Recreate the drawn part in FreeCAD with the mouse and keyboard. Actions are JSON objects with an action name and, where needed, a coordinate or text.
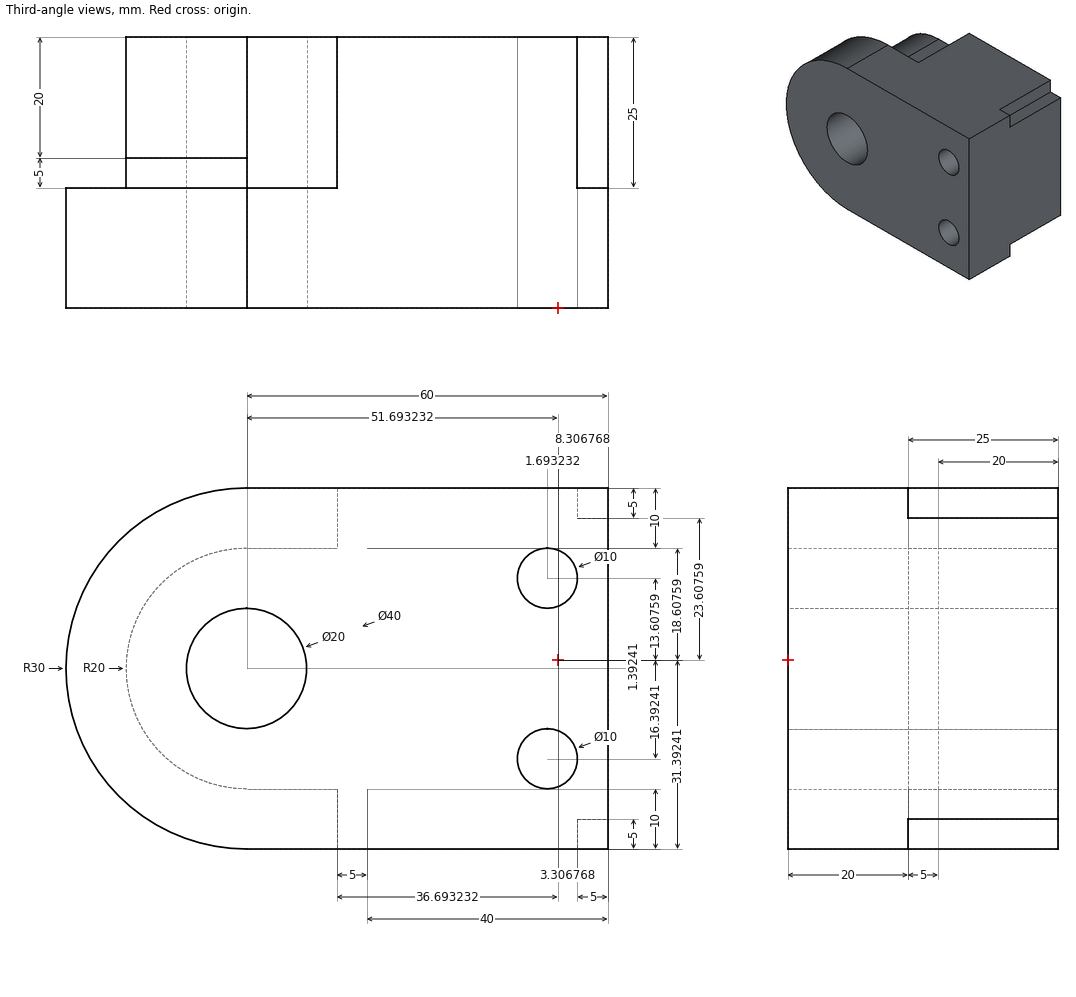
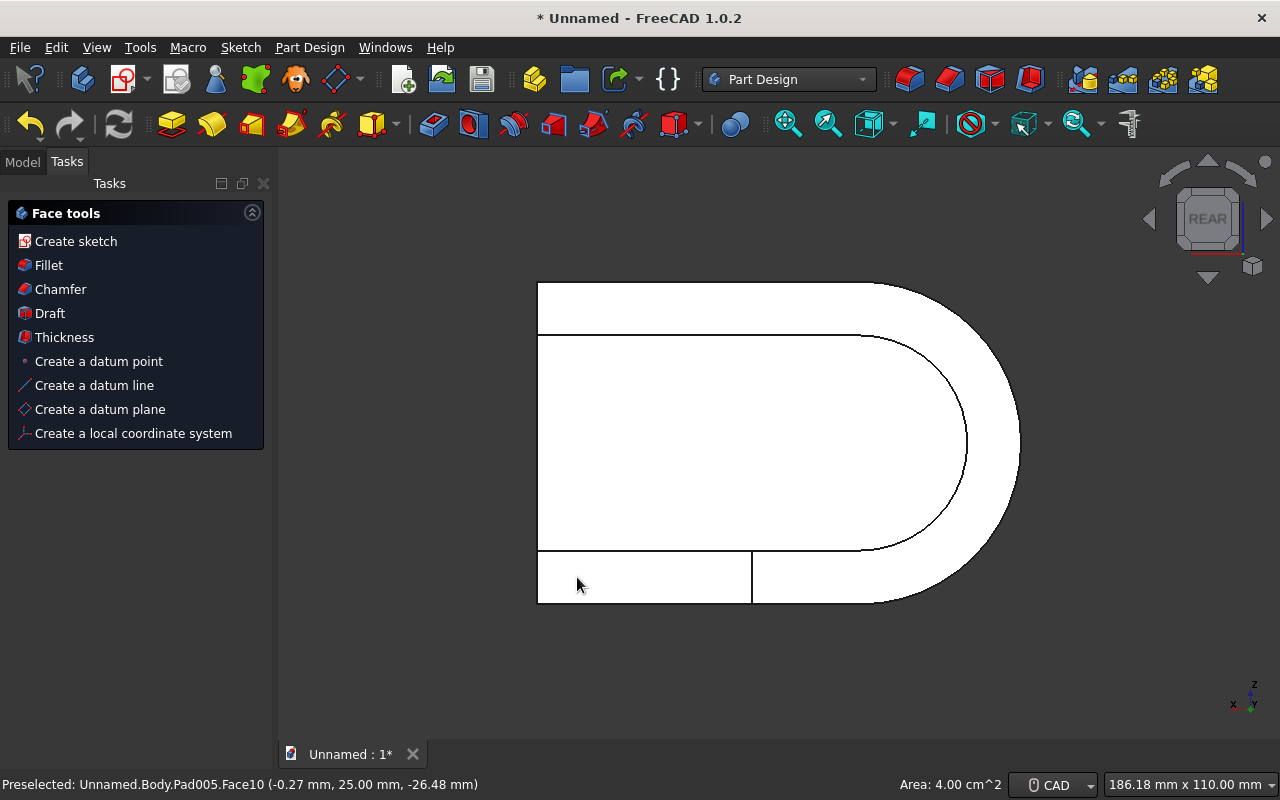
{"action": "left_click", "coordinate": [124, 80]}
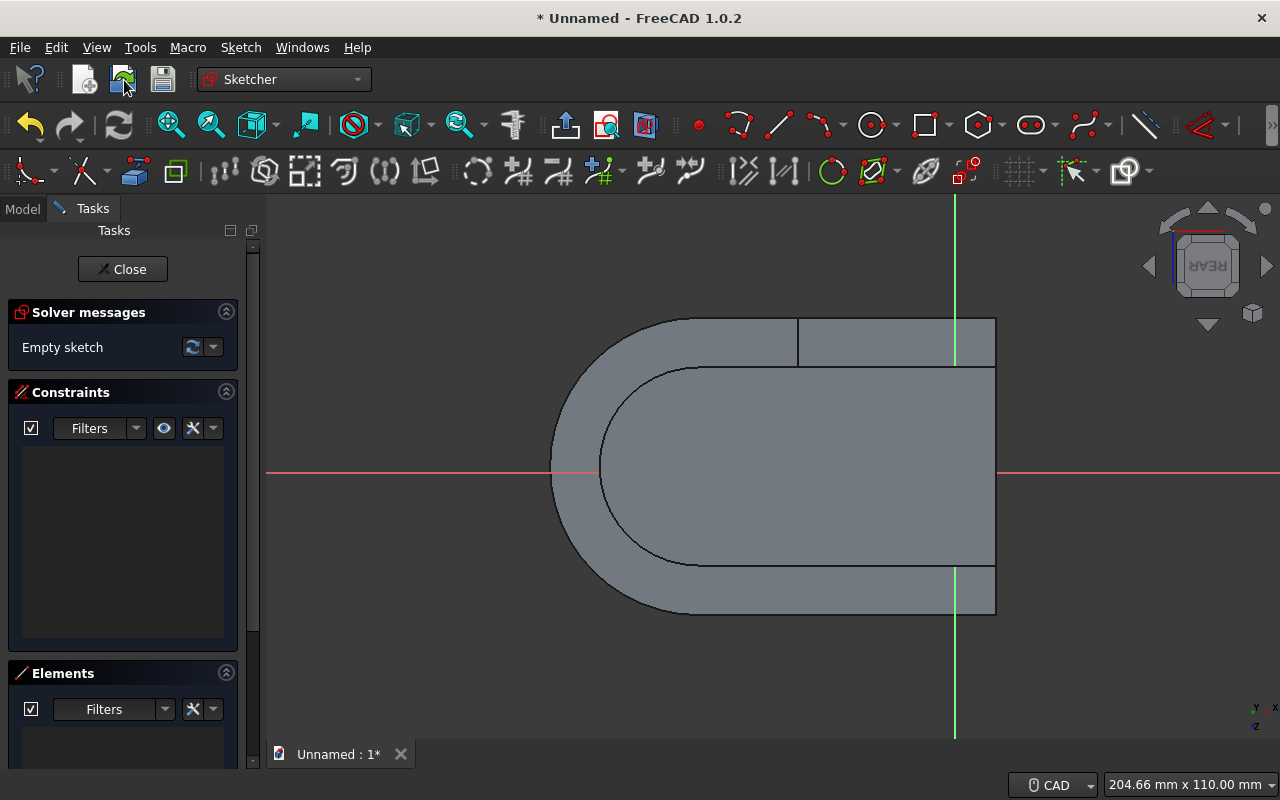
{"action": "left_click", "coordinate": [646, 126]}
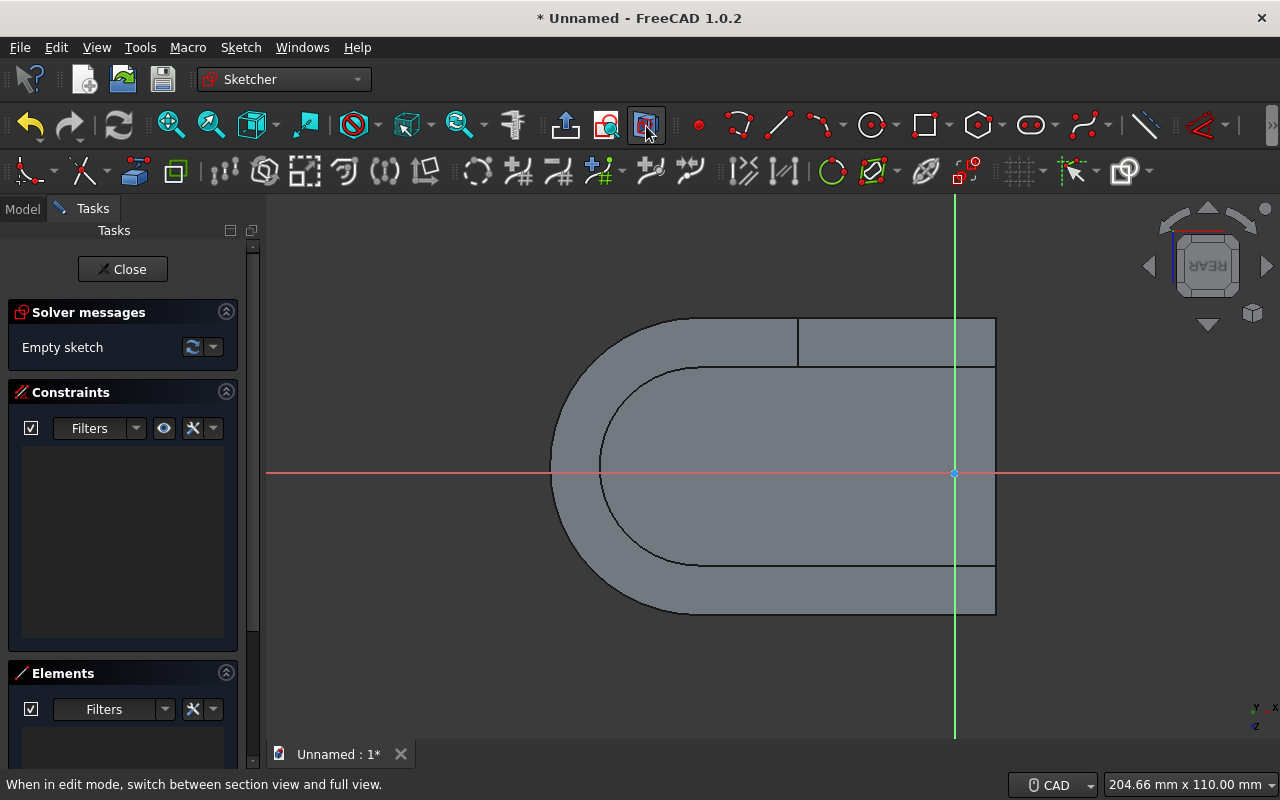
{"action": "scroll", "coordinate": [1054, 338], "scroll_direction": "up", "scroll_amount": 4}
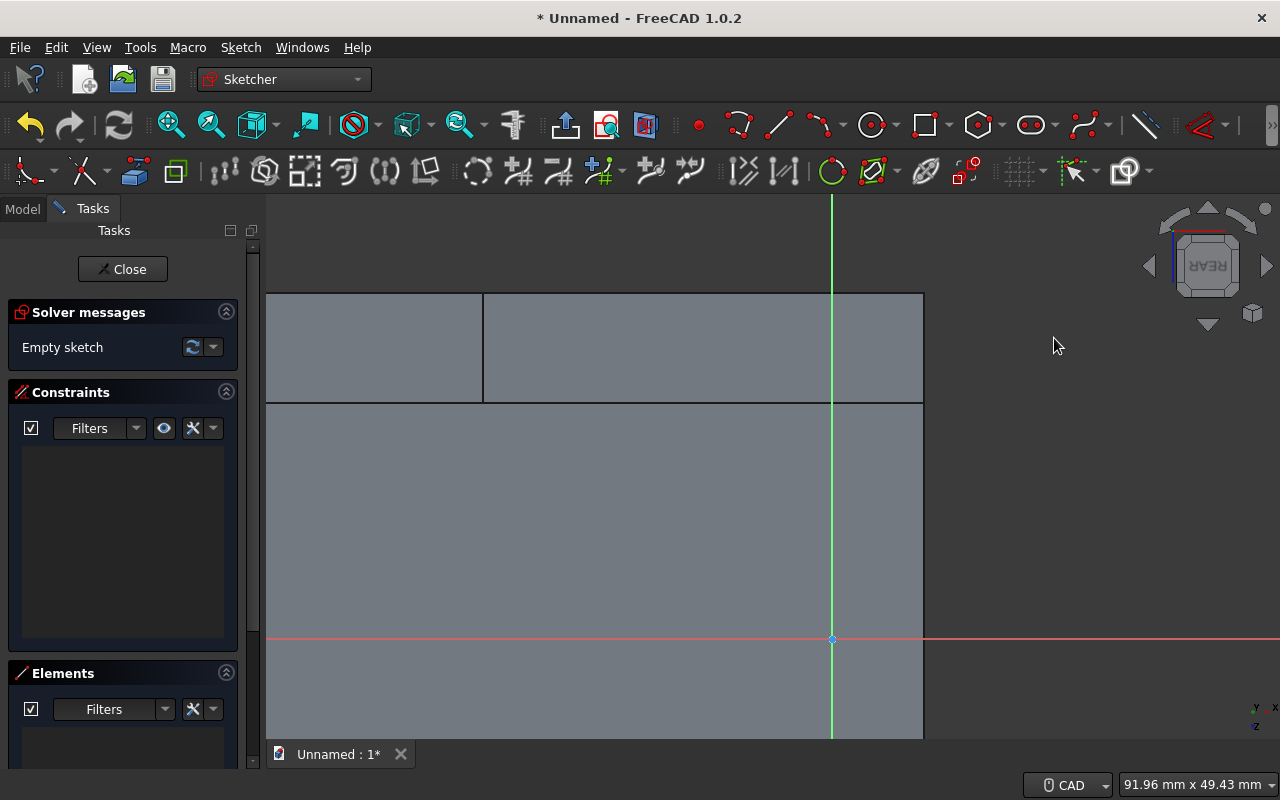
{"action": "key", "text": "g r"}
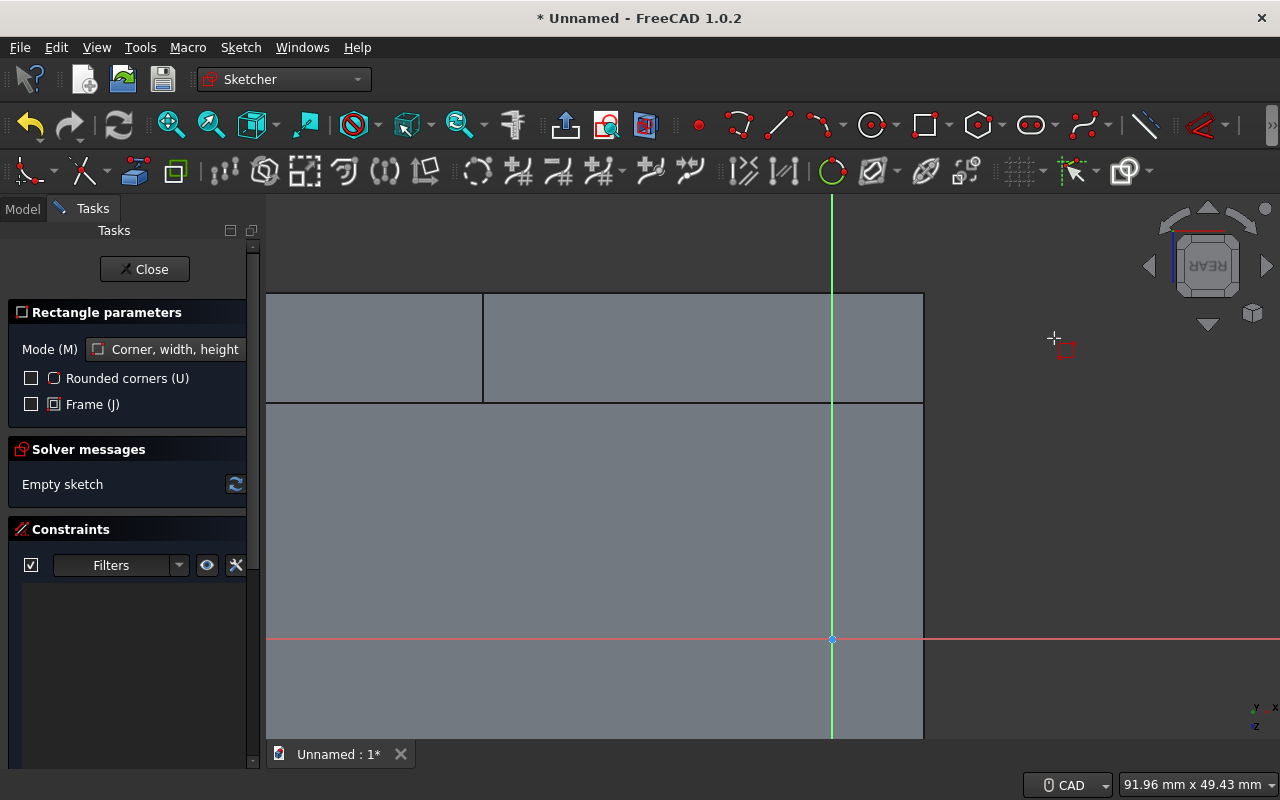
{"action": "left_click", "coordinate": [483, 293]}
{"action": "left_click", "coordinate": [924, 403]}
{"action": "key", "text": "Escape"}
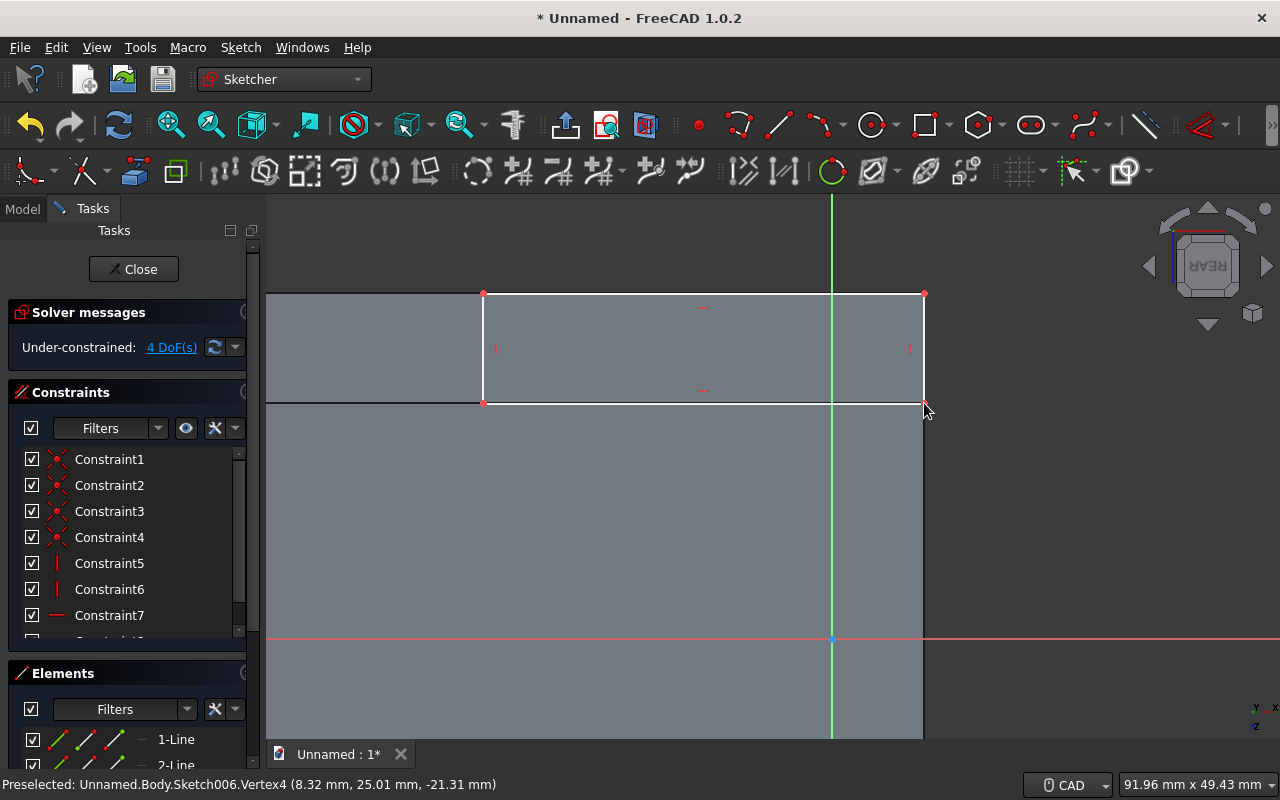
{"action": "left_click", "coordinate": [1200, 126]}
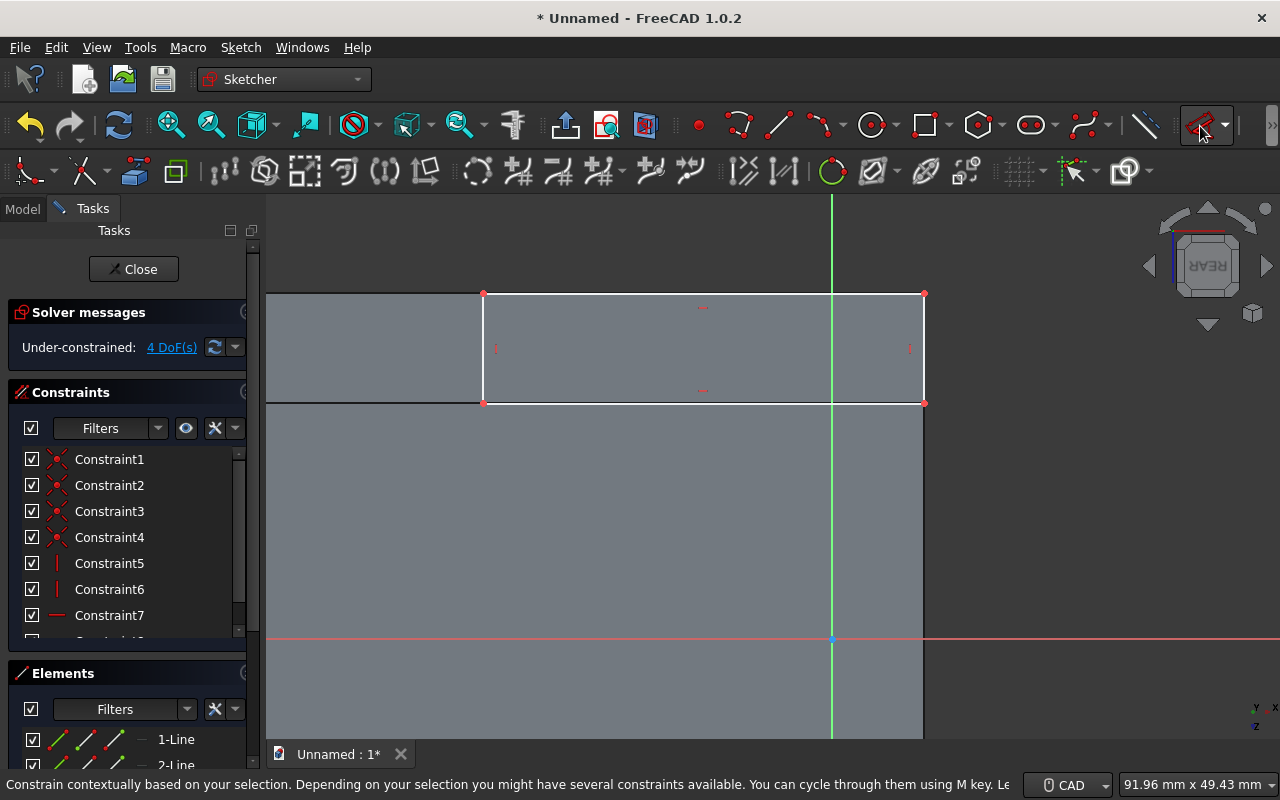
{"action": "left_click", "coordinate": [483, 327]}
{"action": "left_click", "coordinate": [449, 349]}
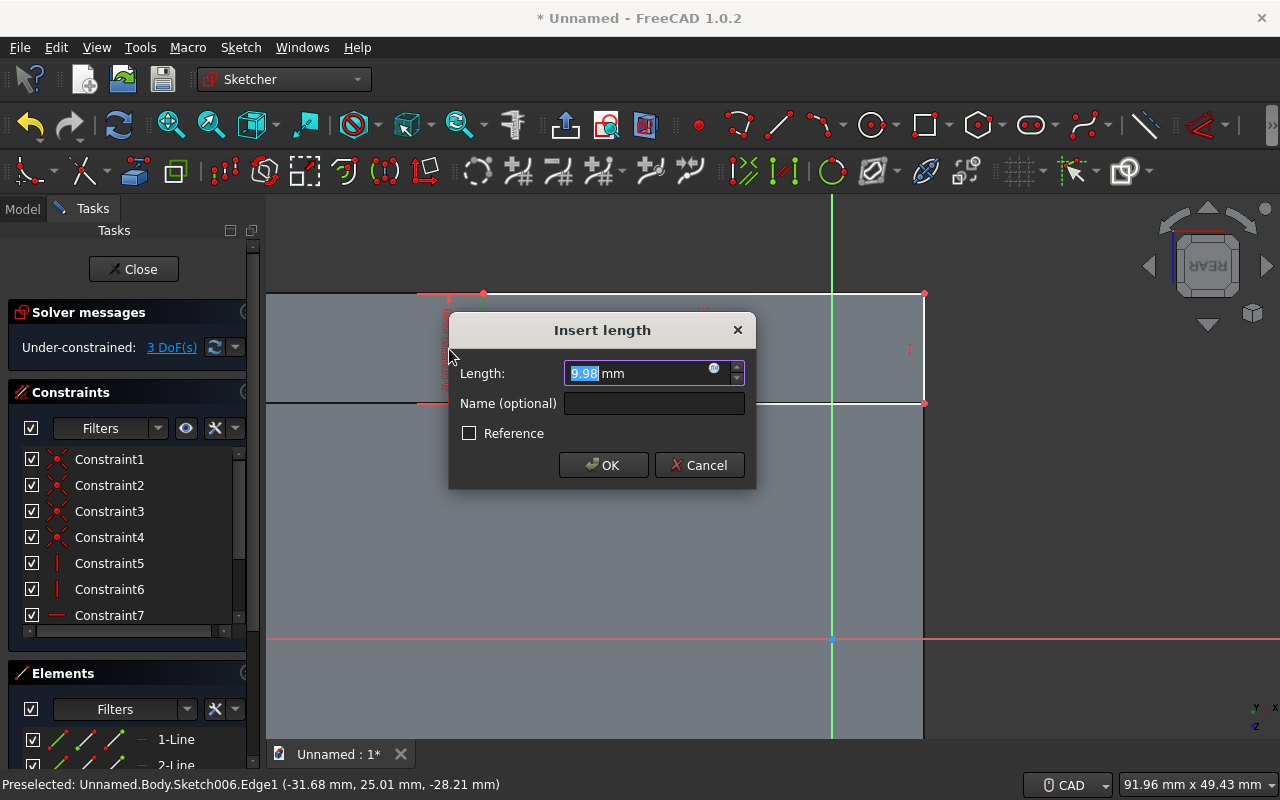
{"action": "type", "text": "10"}
{"action": "key", "text": "Return"}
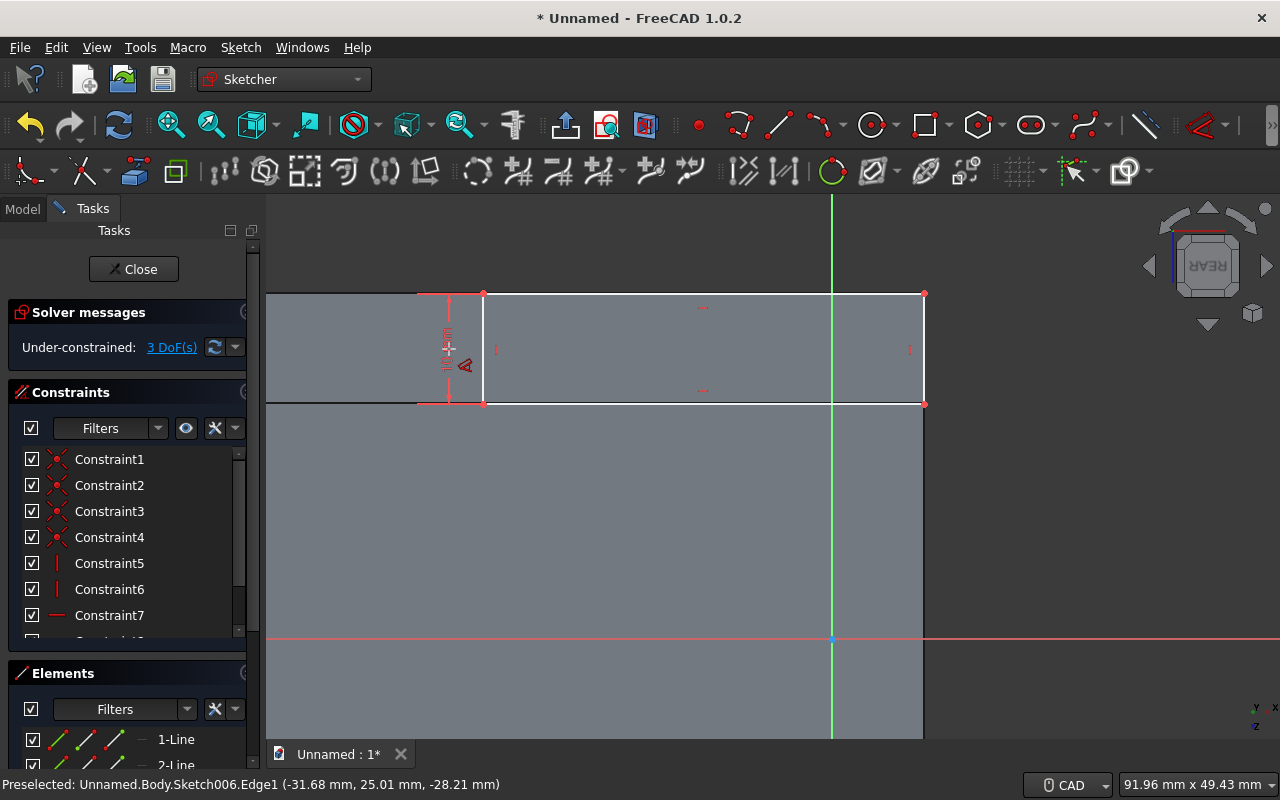
{"action": "left_click", "coordinate": [615, 404]}
{"action": "left_click", "coordinate": [703, 370]}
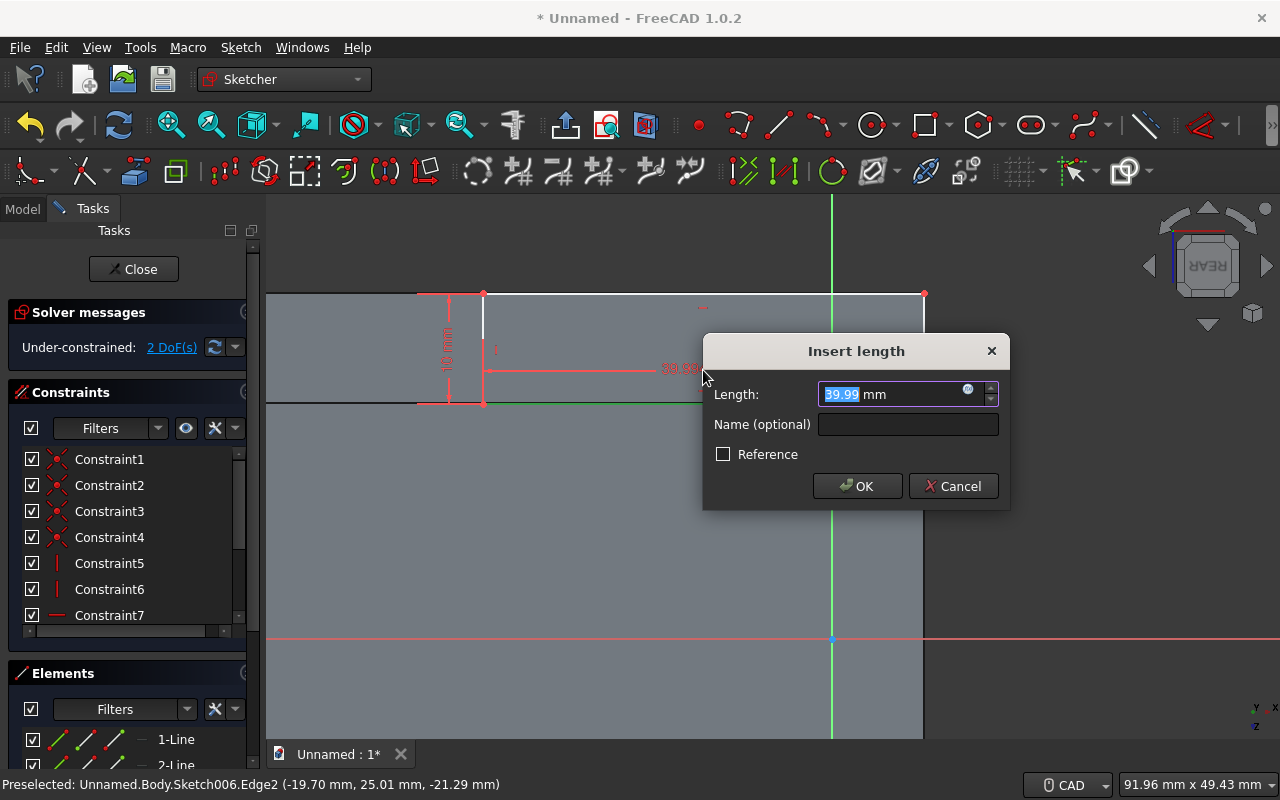
{"action": "type", "text": "40"}
{"action": "key", "text": "Return"}